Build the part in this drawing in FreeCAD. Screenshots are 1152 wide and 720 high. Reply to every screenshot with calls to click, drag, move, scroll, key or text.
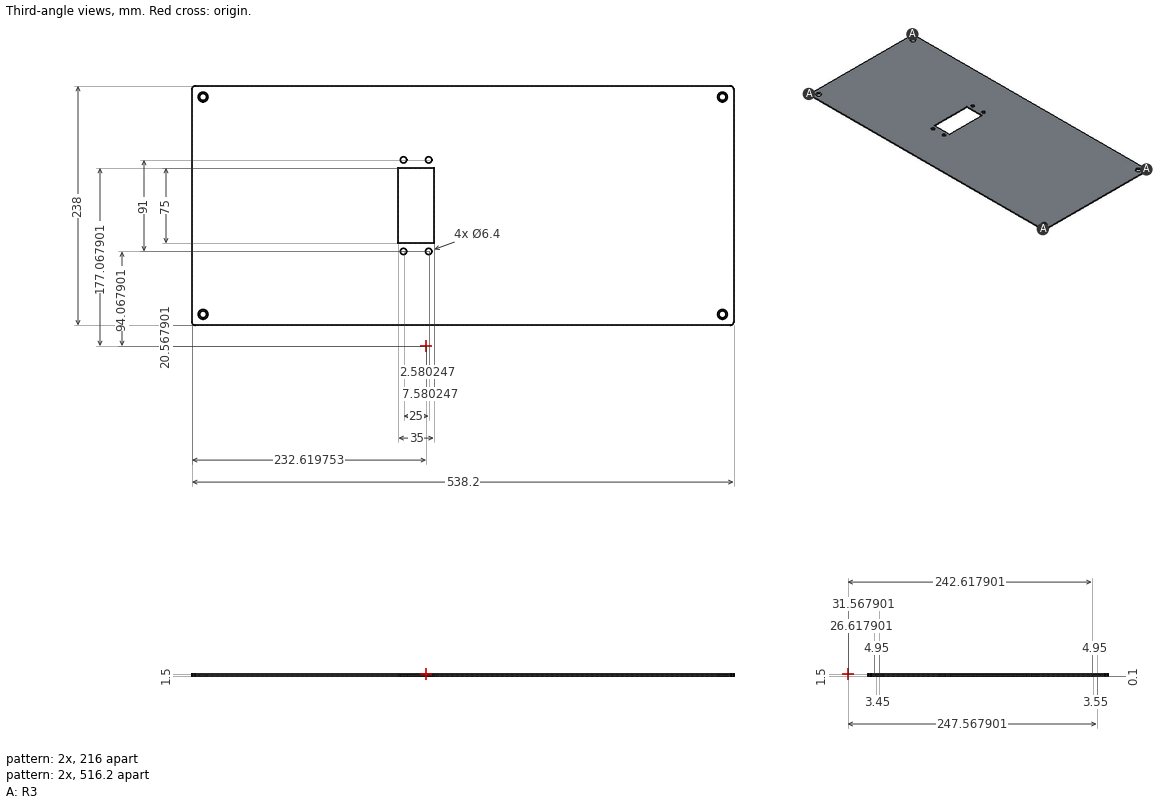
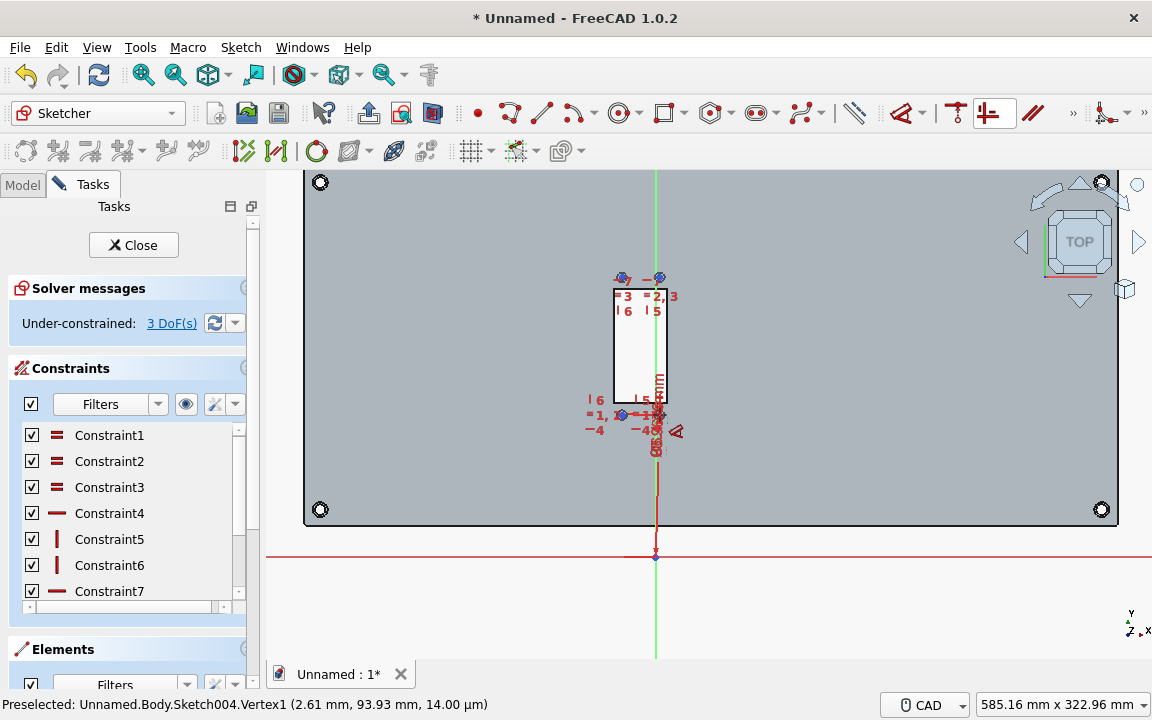
click(622, 415)
click(641, 449)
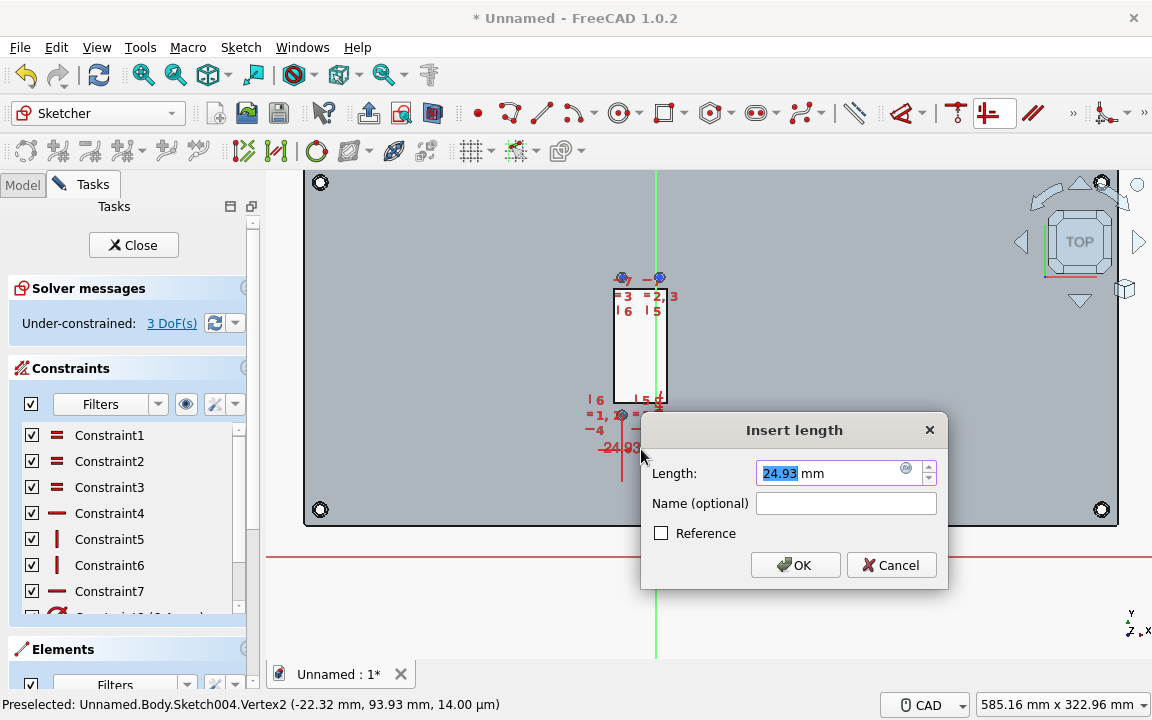
text(25)
key(Return)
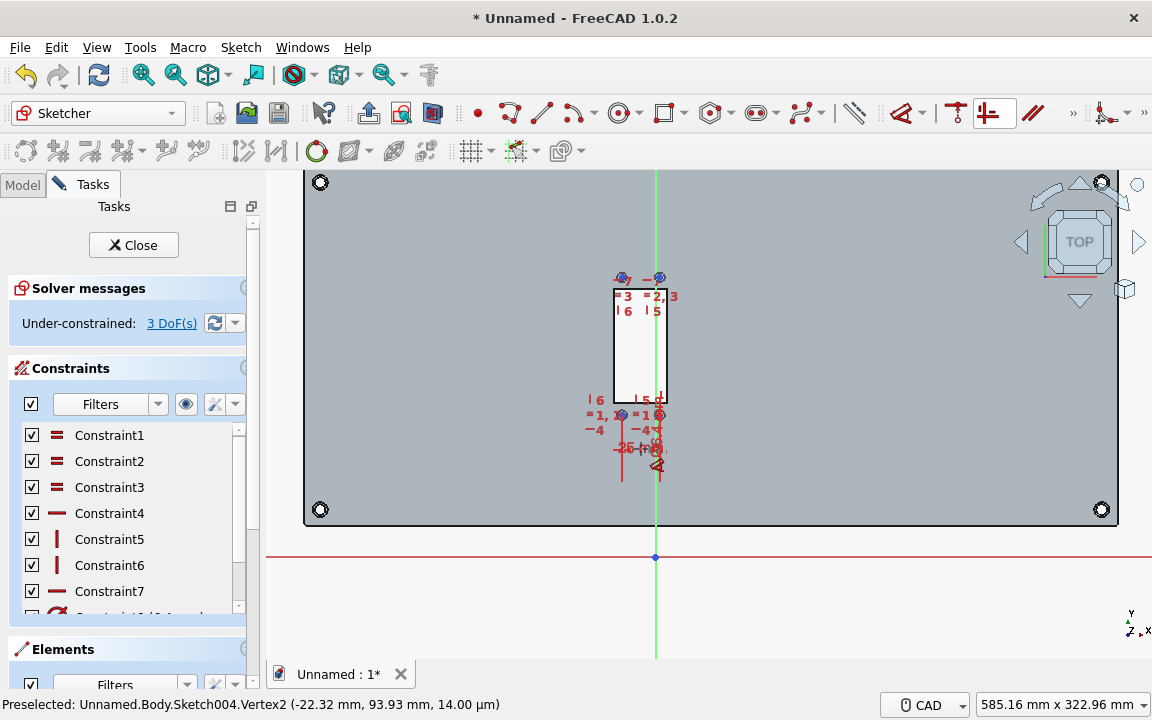
click(660, 415)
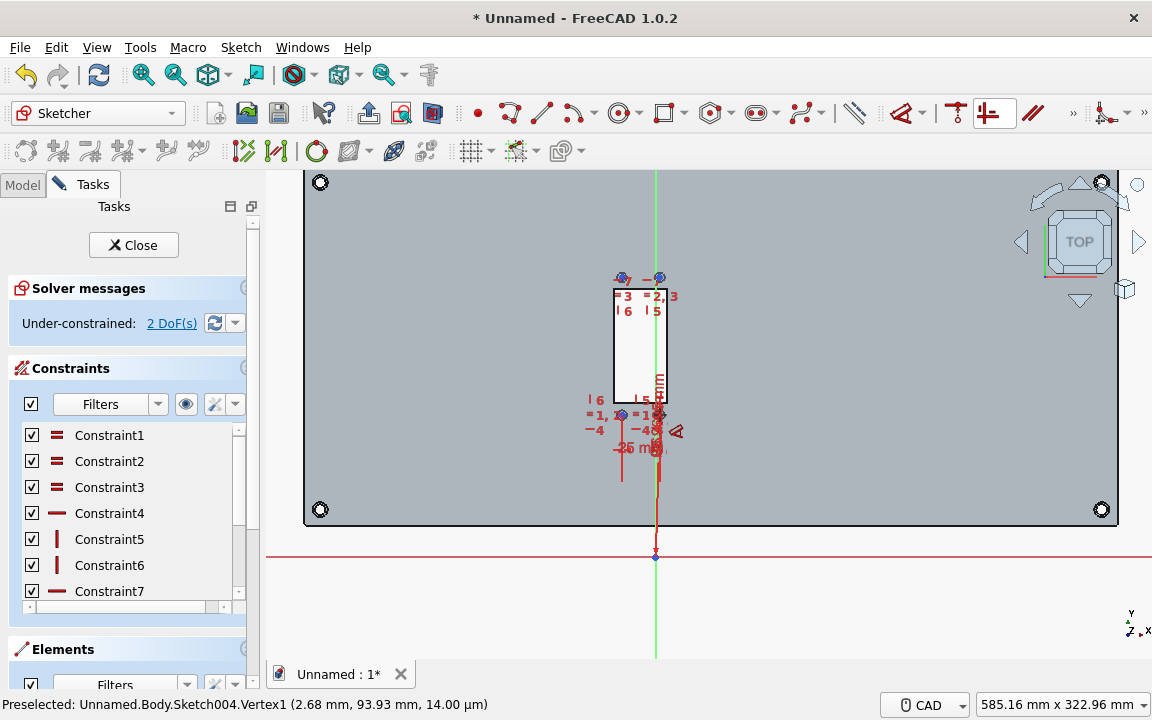
click(660, 277)
click(694, 346)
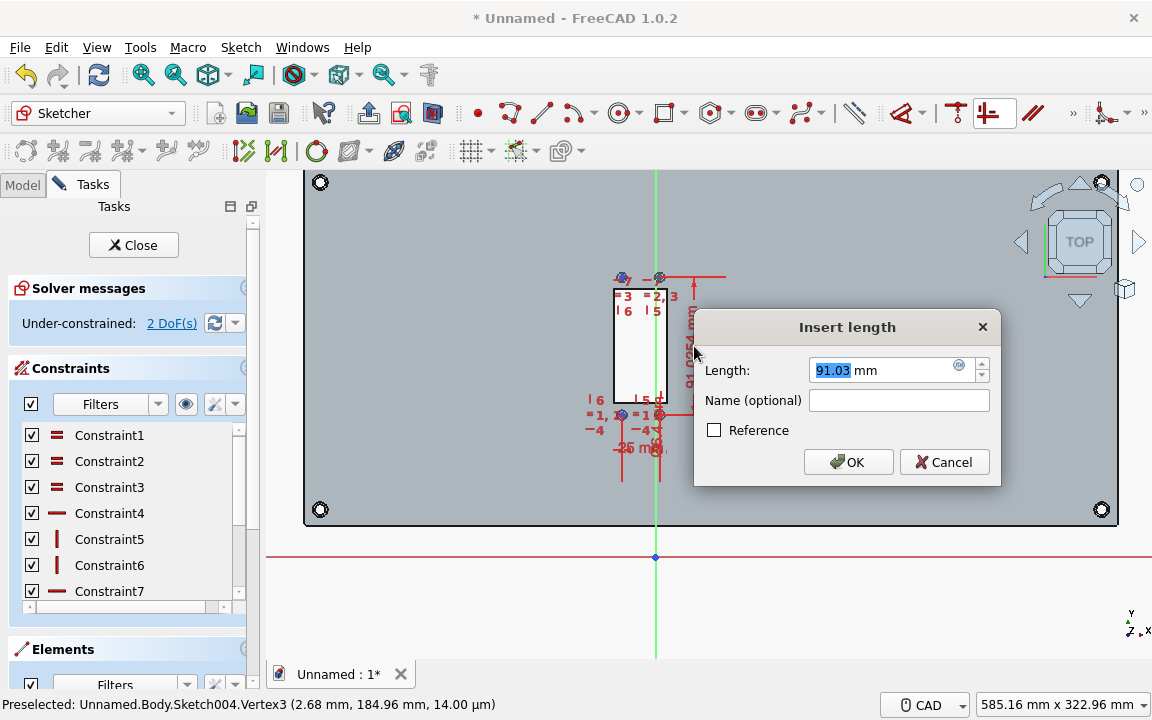
text(91)
key(Return)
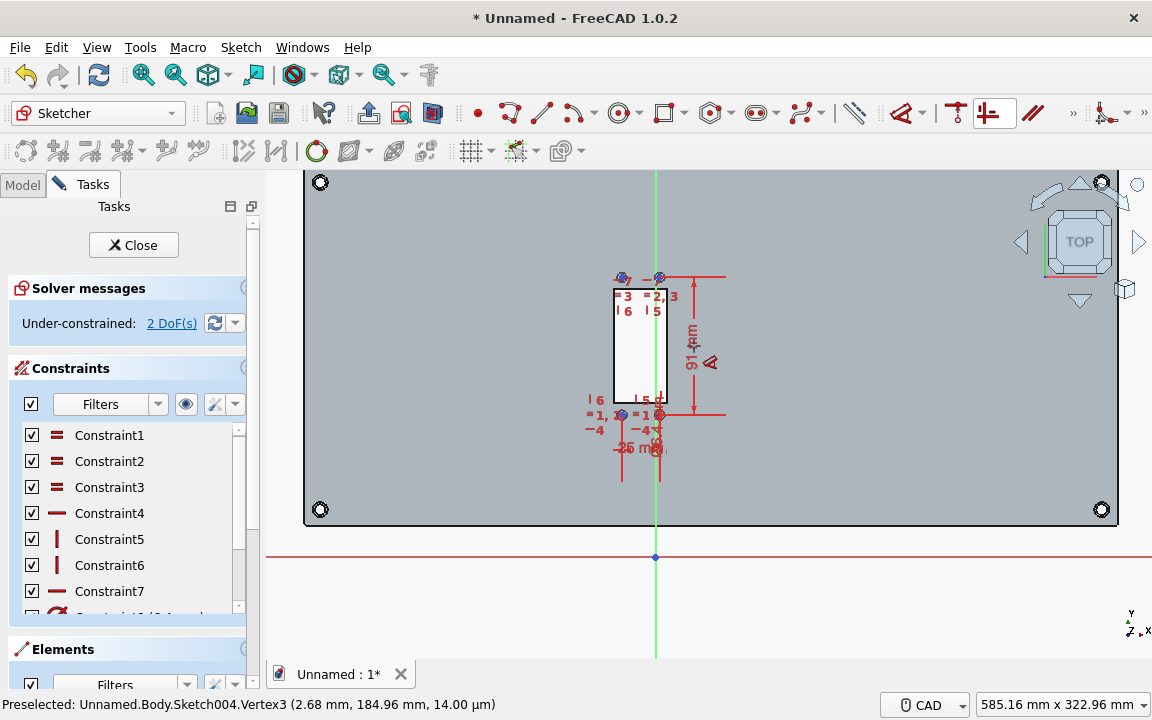
scroll(660, 415, up, 12)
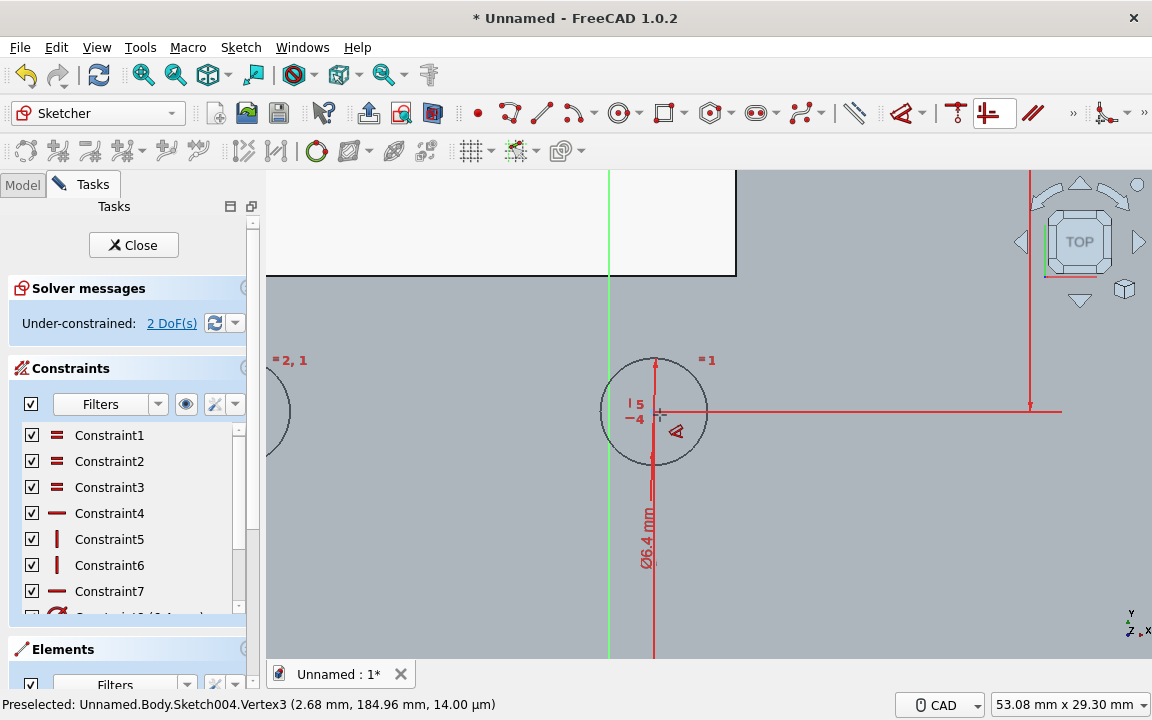
click(654, 412)
click(642, 378)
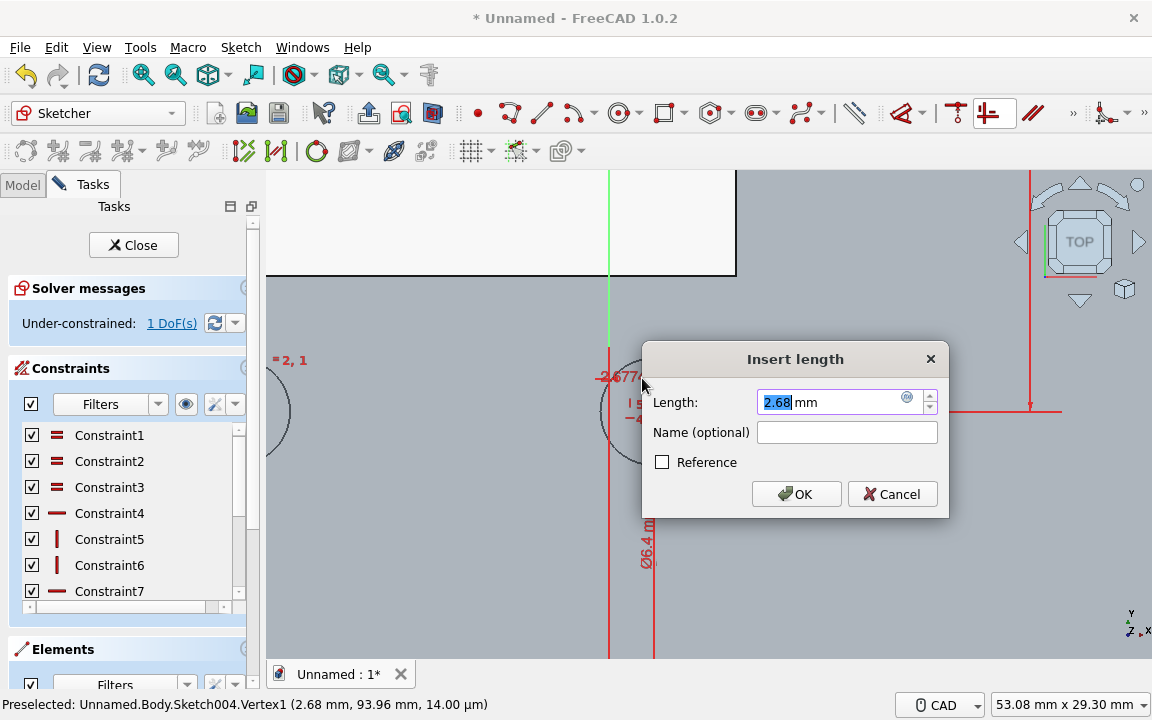
text(2.580247)
key(Return)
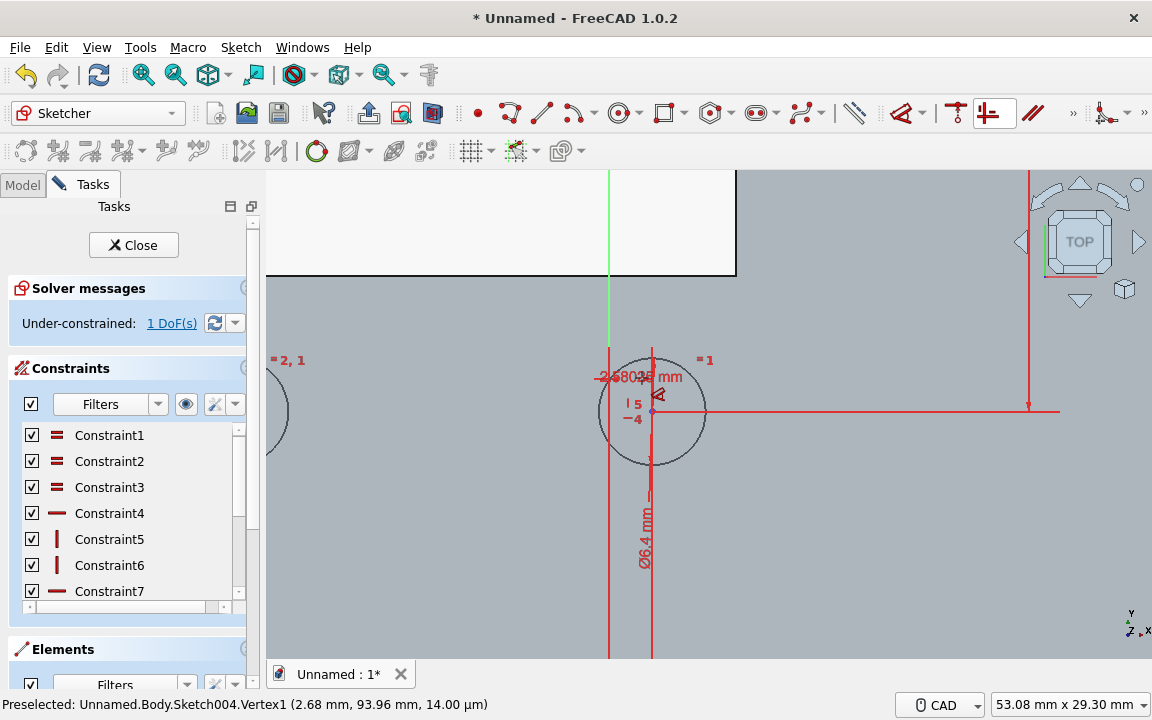
scroll(660, 415, down, 12)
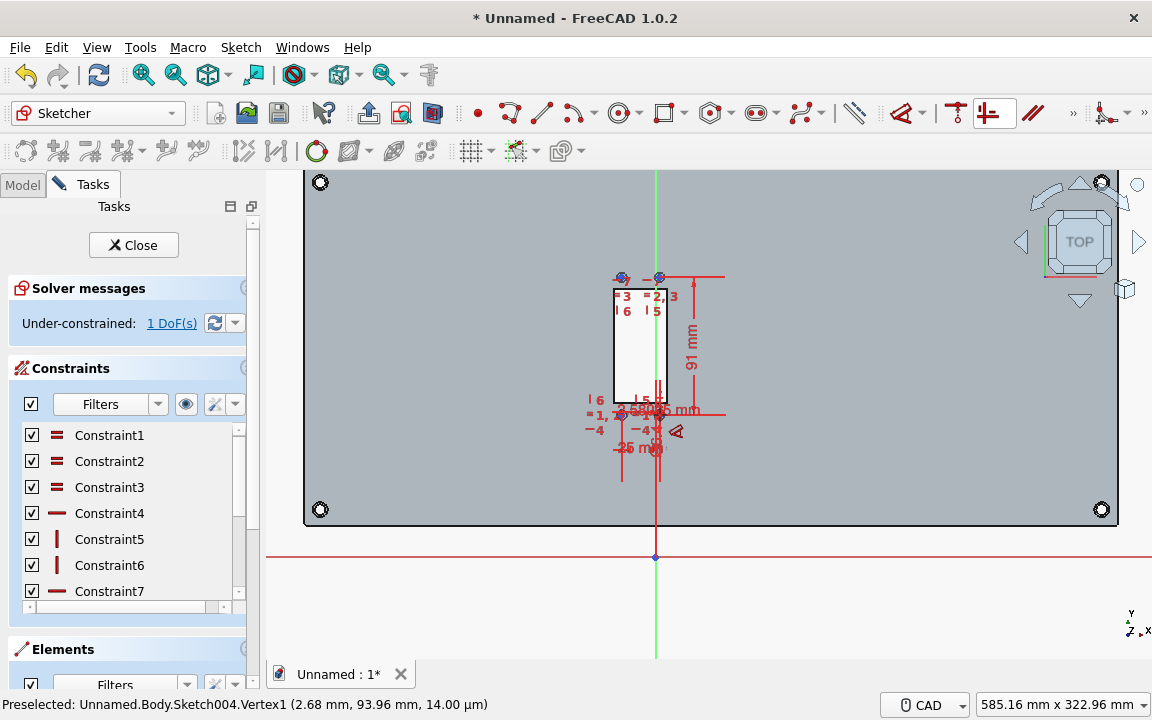
click(660, 415)
click(694, 486)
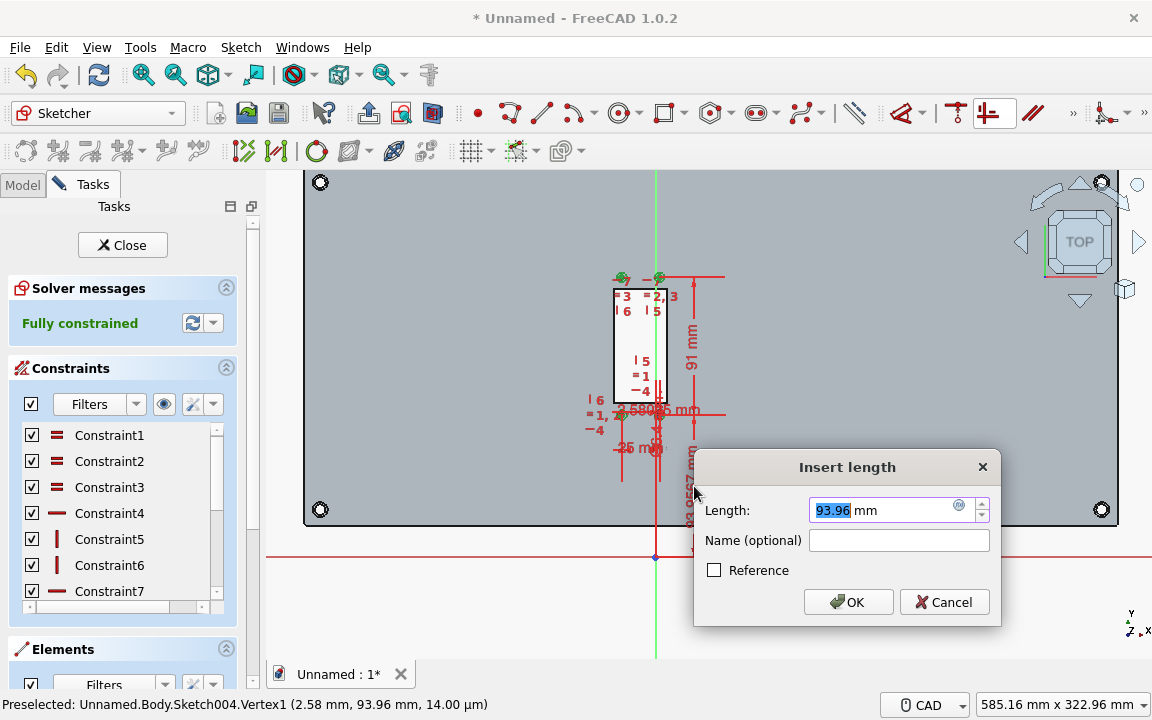
text(94.067901)
key(Return)
key(Escape)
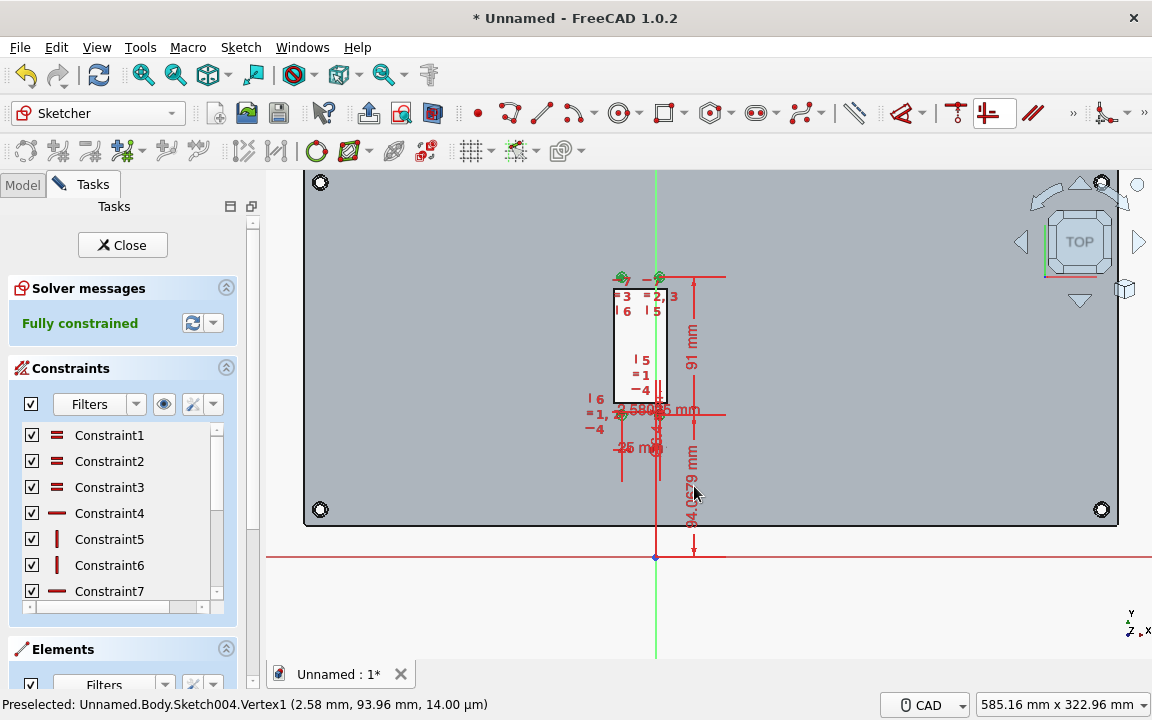
click(123, 245)